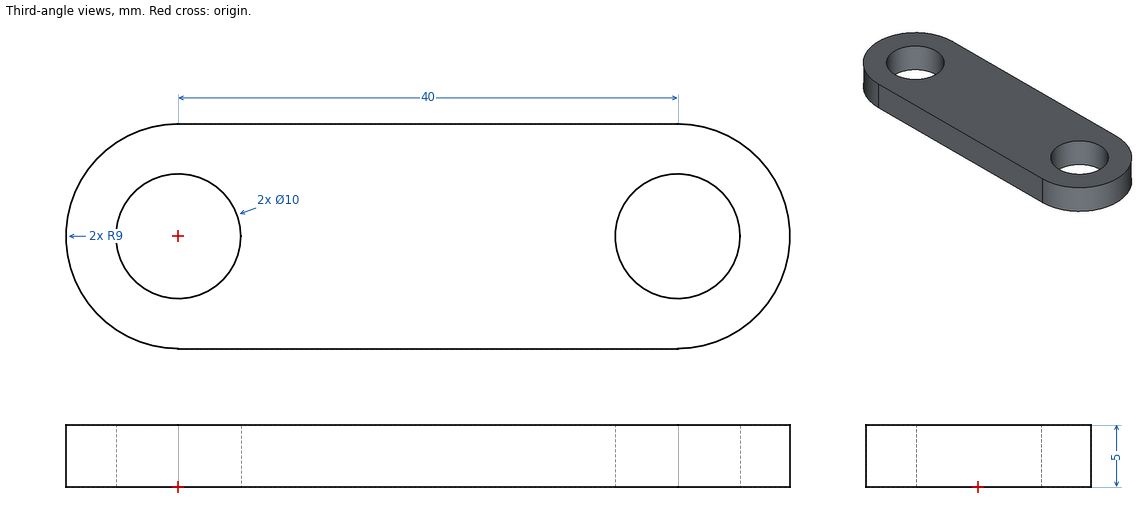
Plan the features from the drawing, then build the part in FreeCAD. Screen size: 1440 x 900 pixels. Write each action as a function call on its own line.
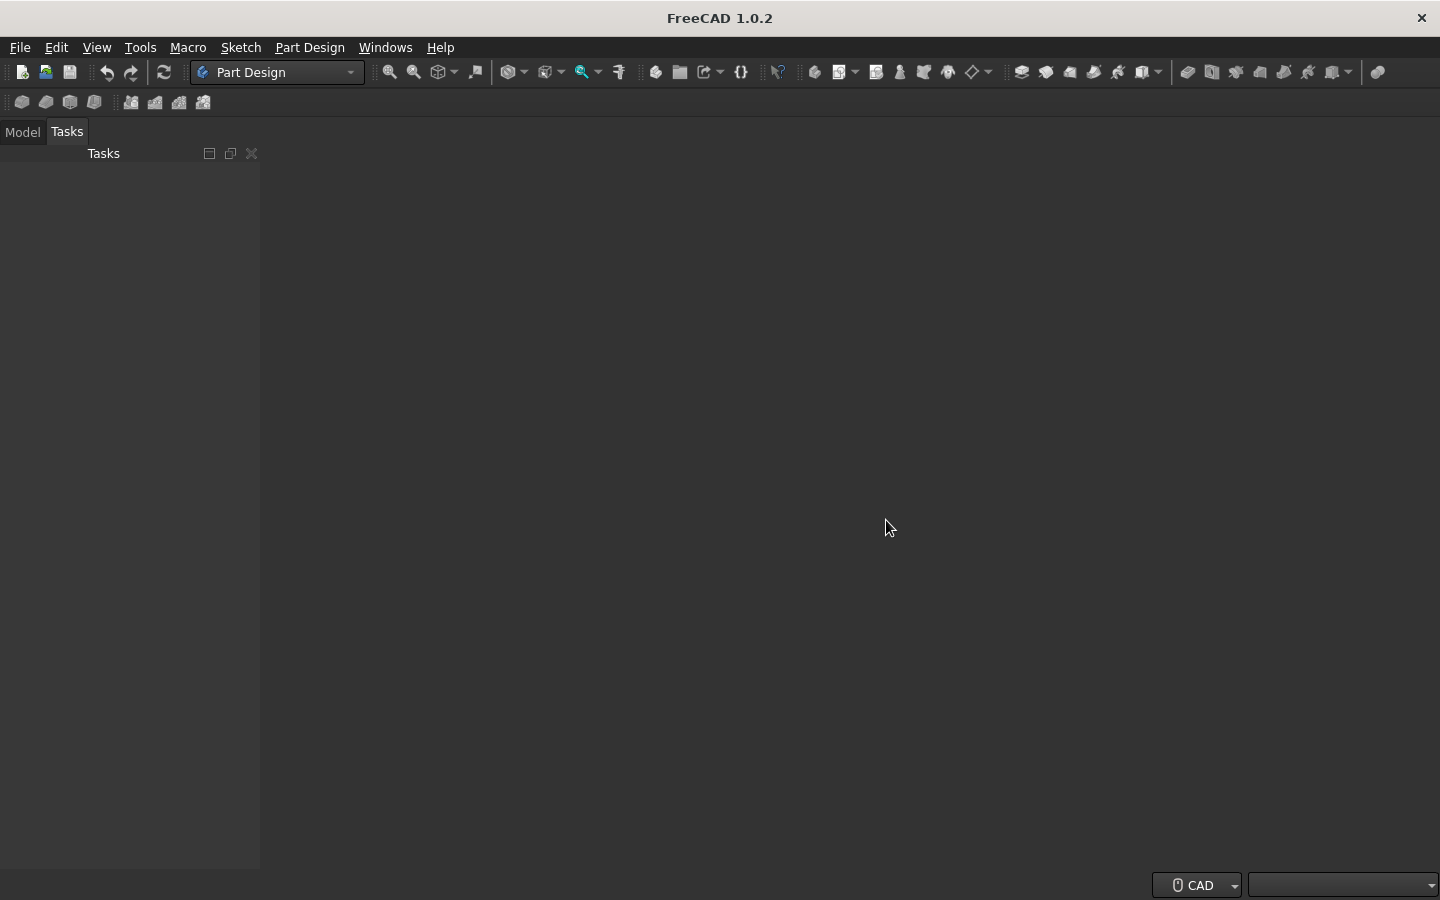
click(22, 72)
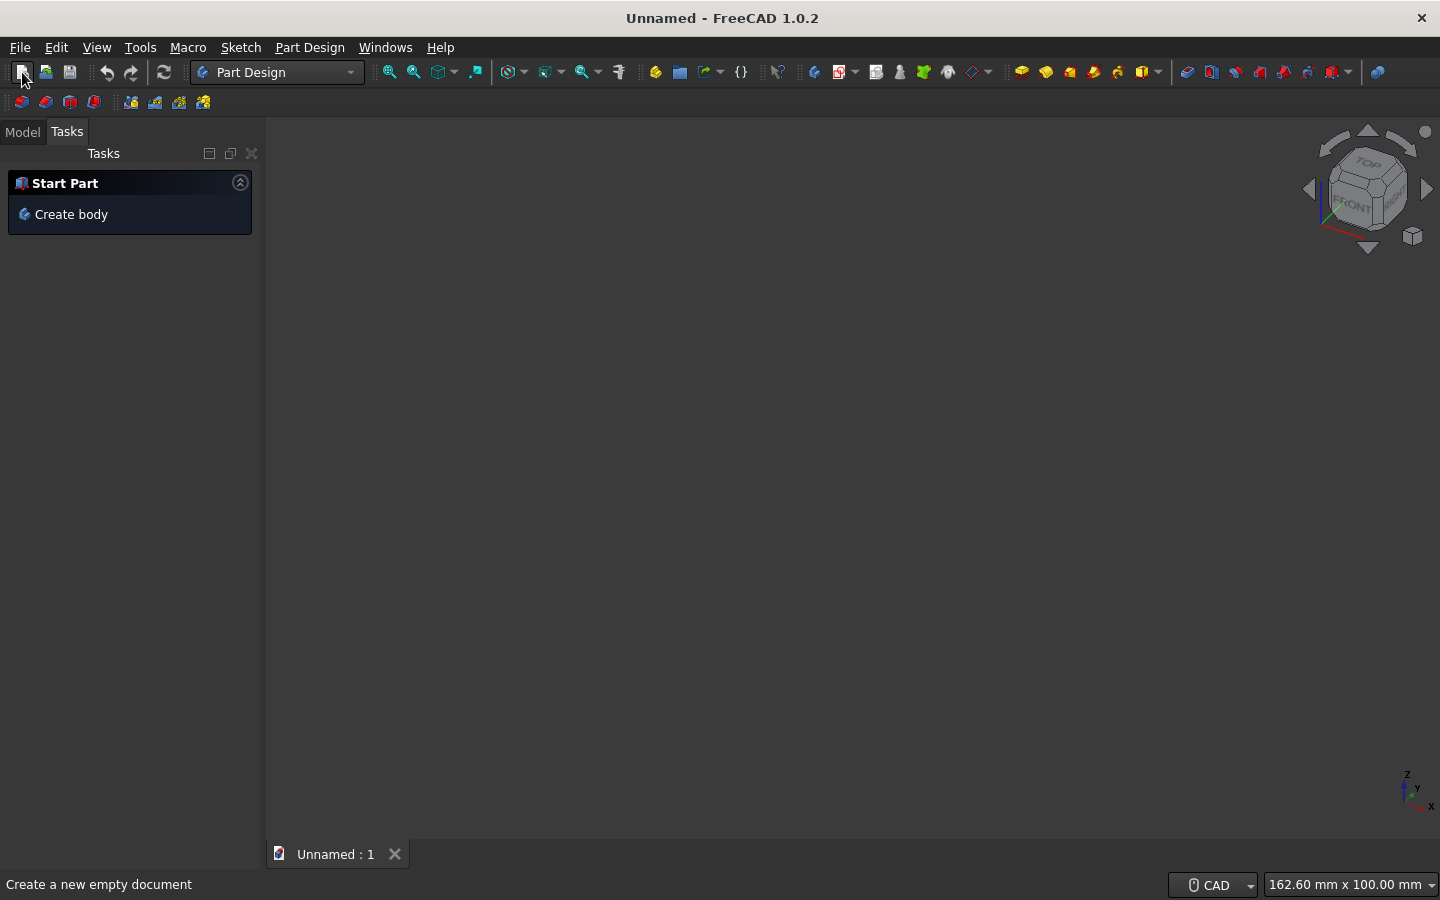
click(840, 72)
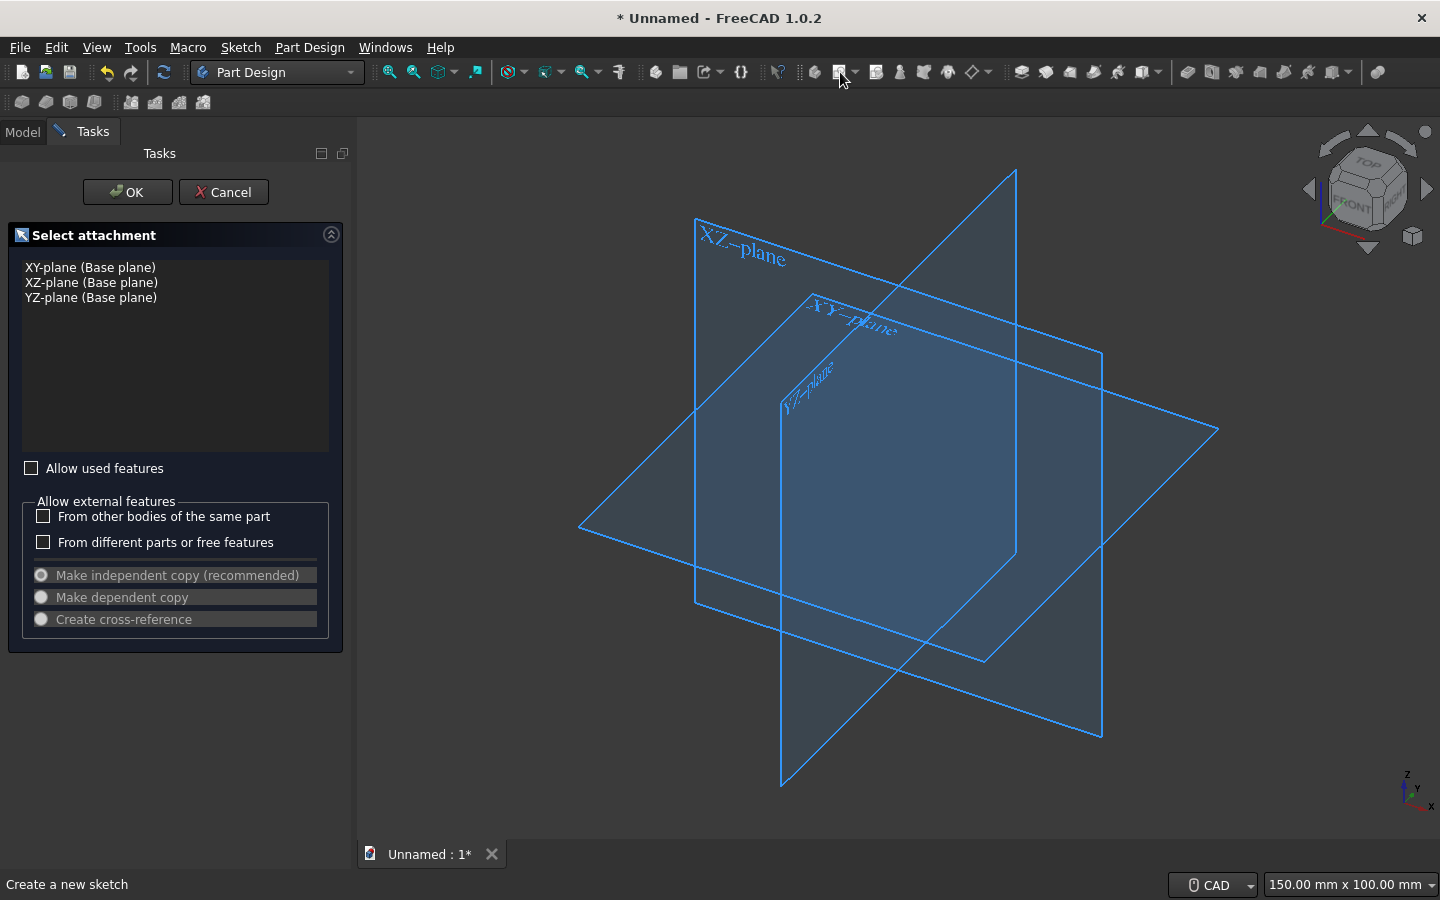
click(82, 268)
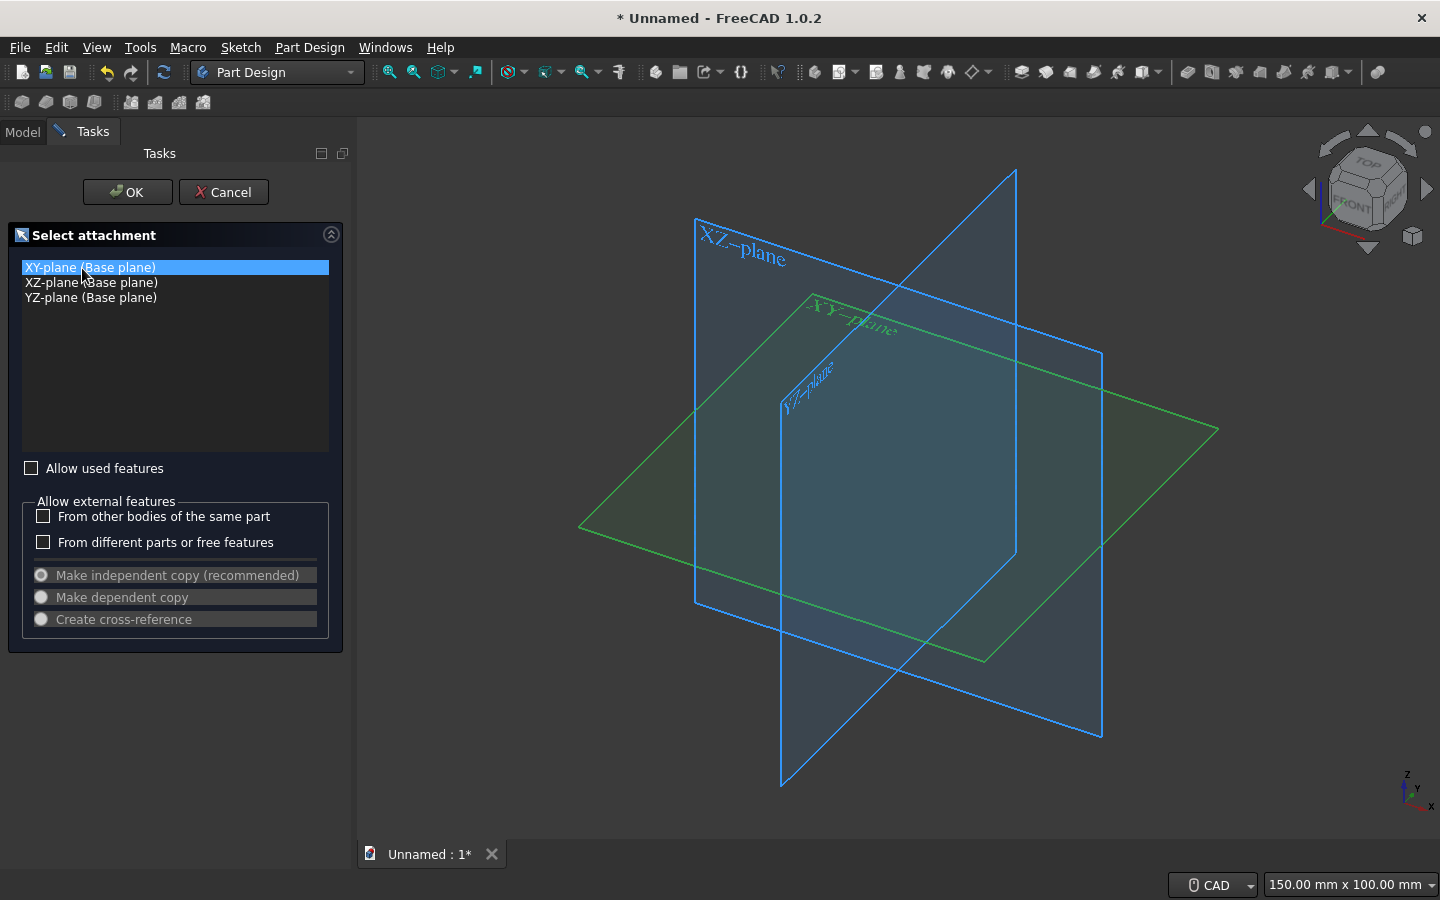
click(128, 192)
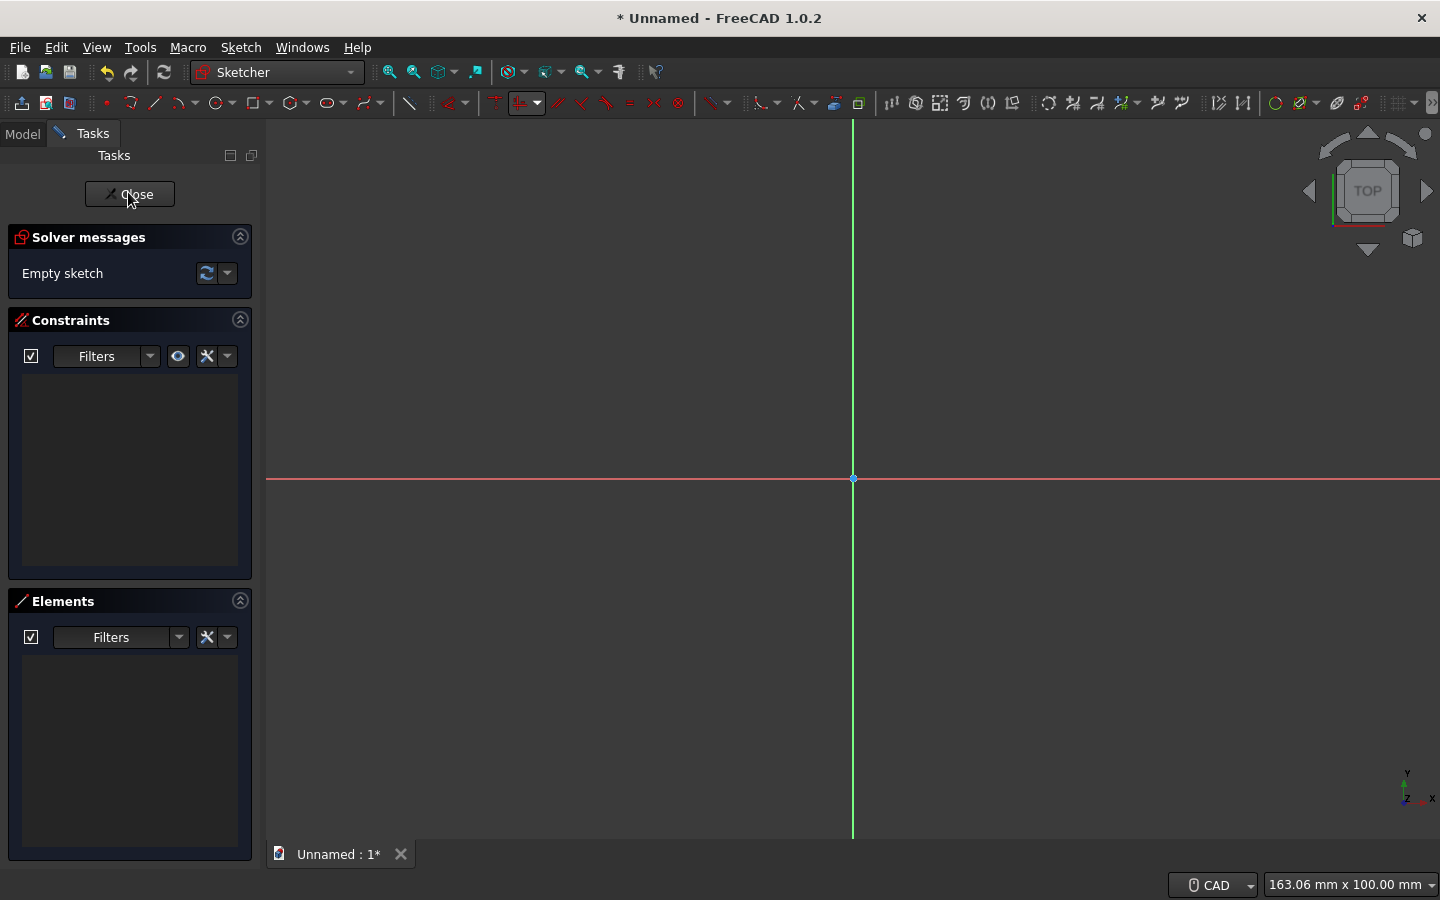
scroll(1255, 479, up, 3)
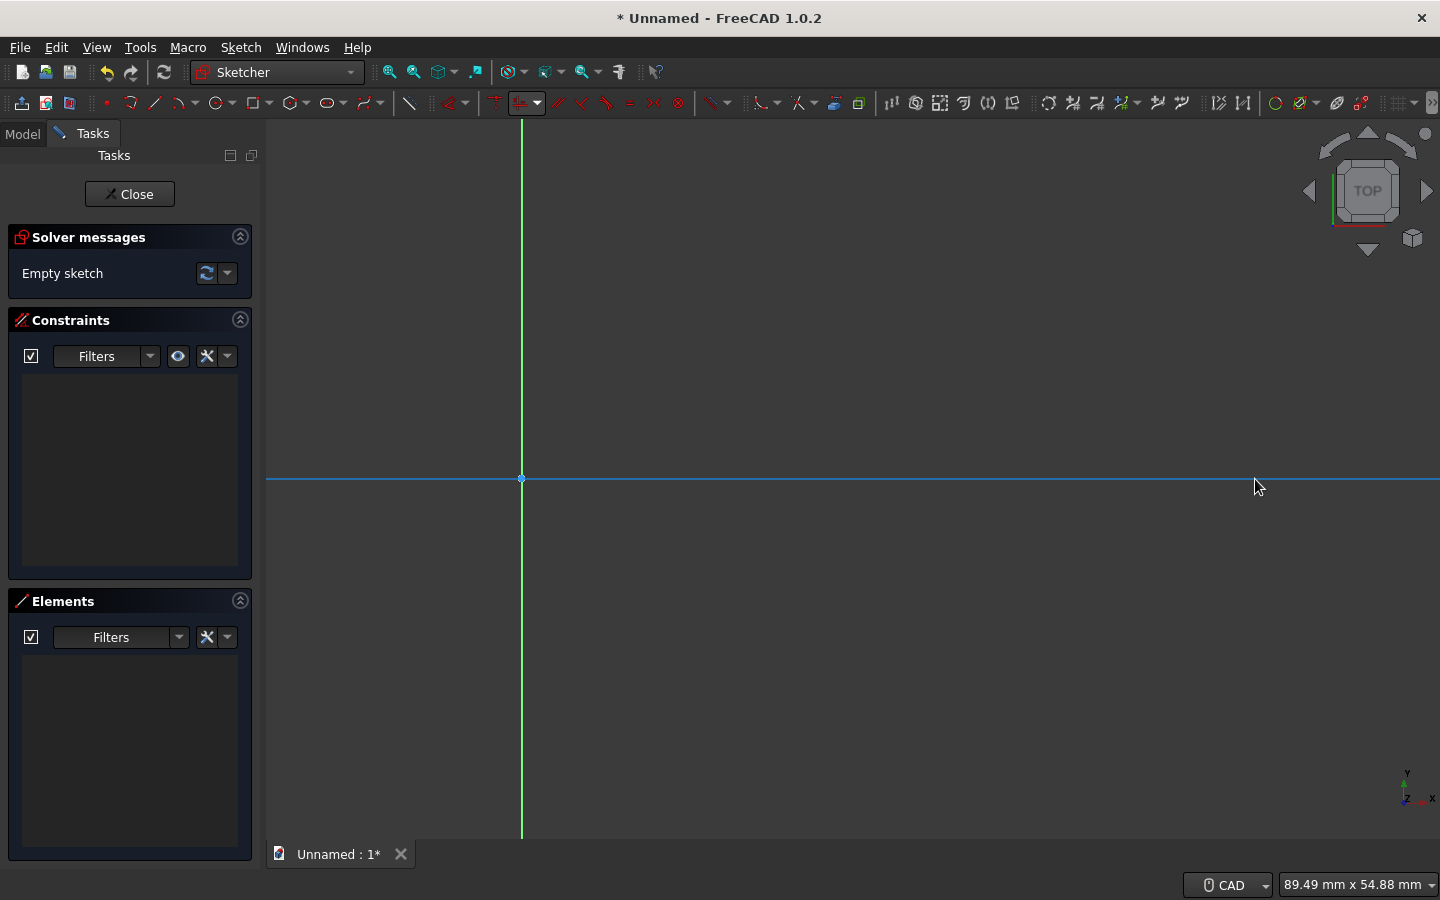
key(g)
key(s)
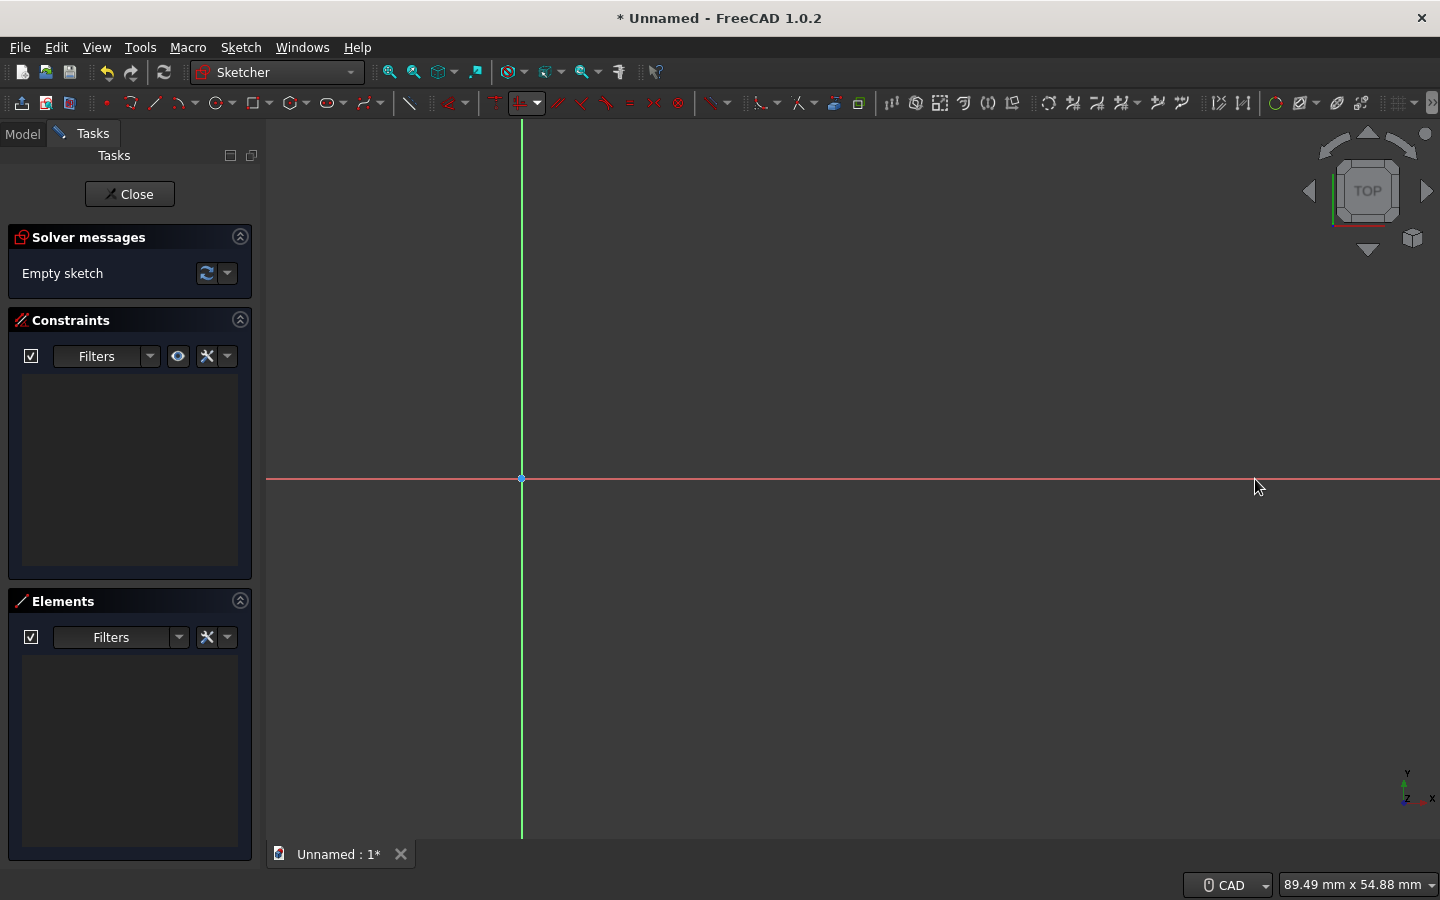
click(522, 479)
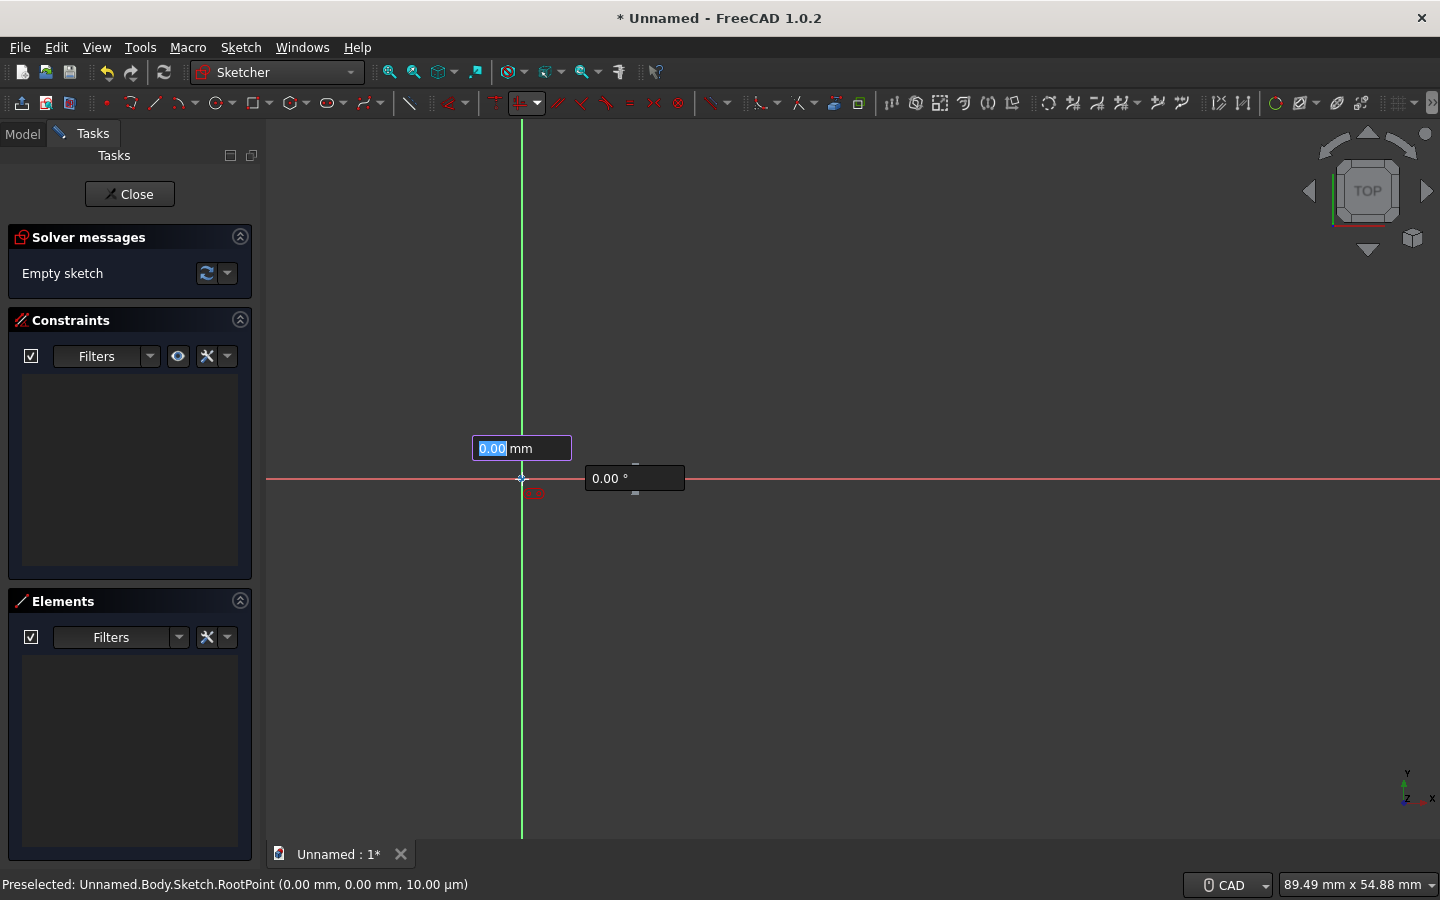
click(1047, 470)